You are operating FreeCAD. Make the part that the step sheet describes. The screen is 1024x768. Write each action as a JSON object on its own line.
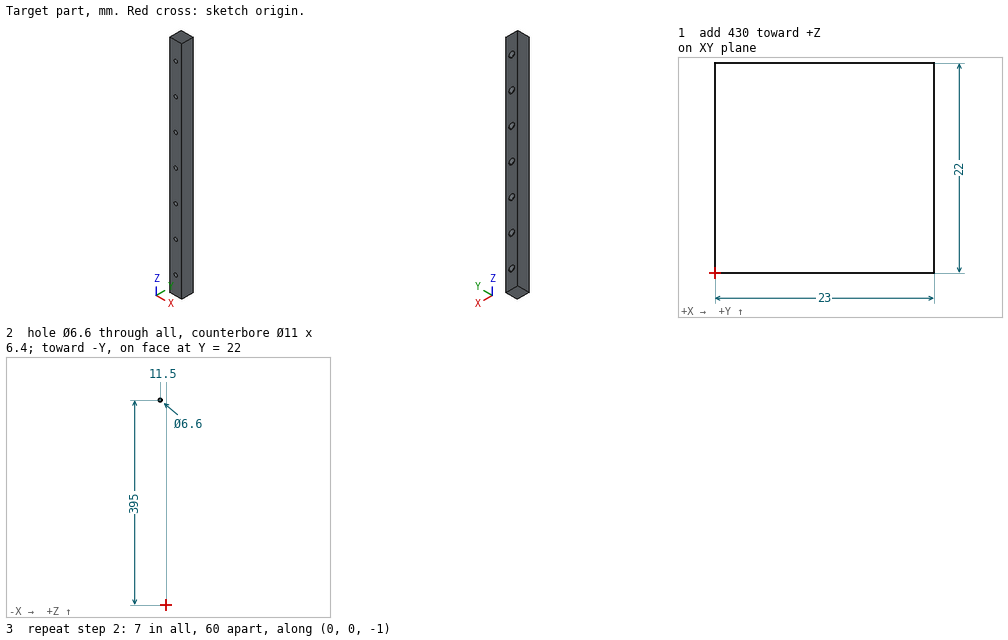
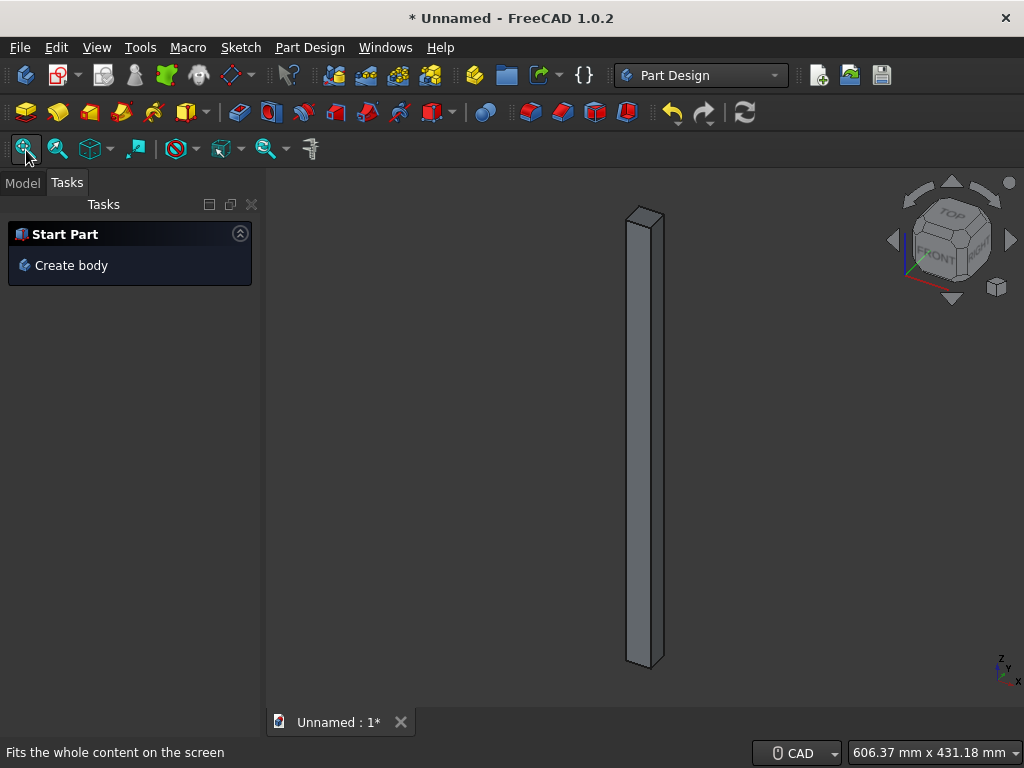
{"action": "key", "text": "4"}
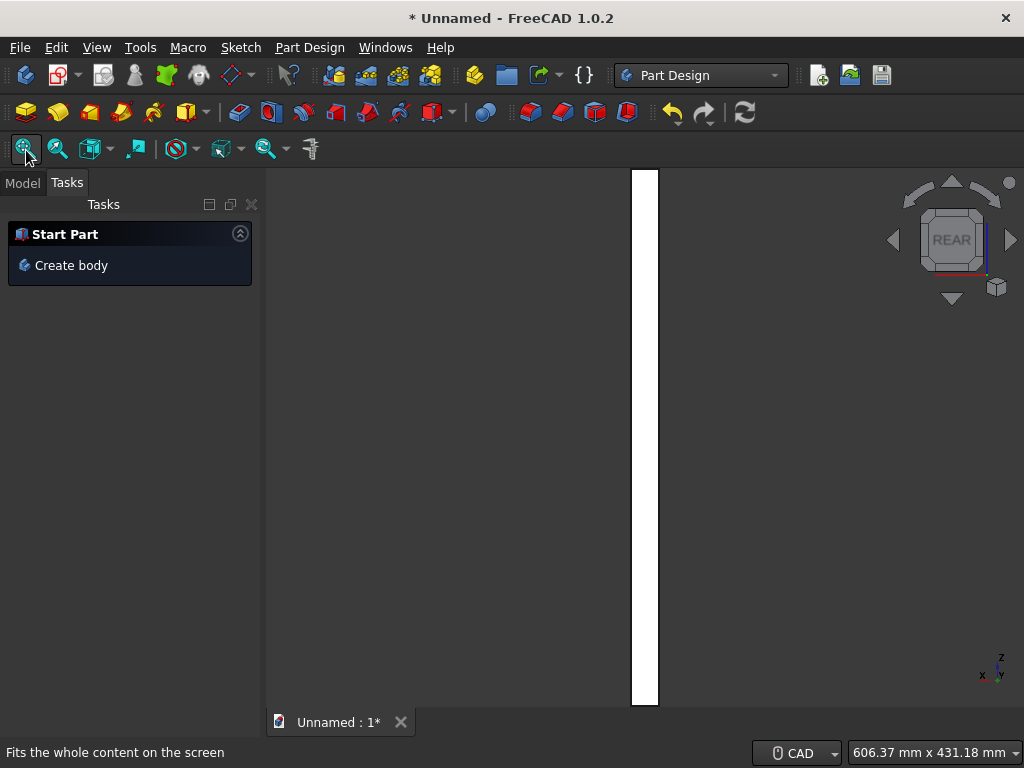
{"action": "left_click", "coordinate": [645, 206]}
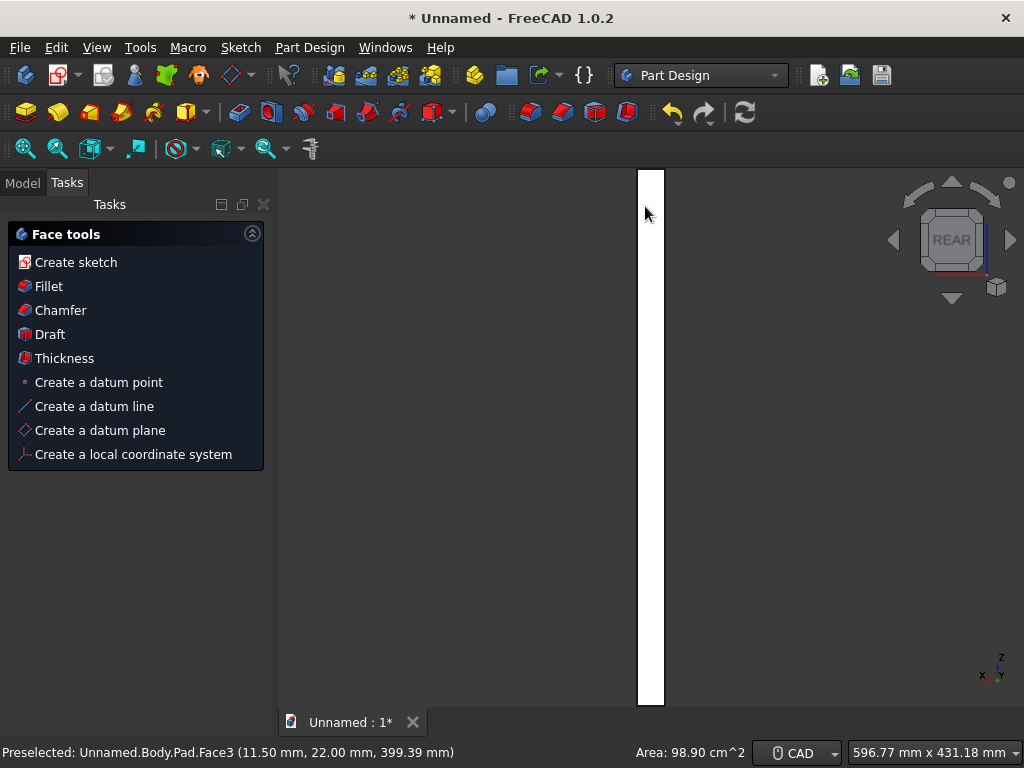
{"action": "left_click", "coordinate": [58, 76]}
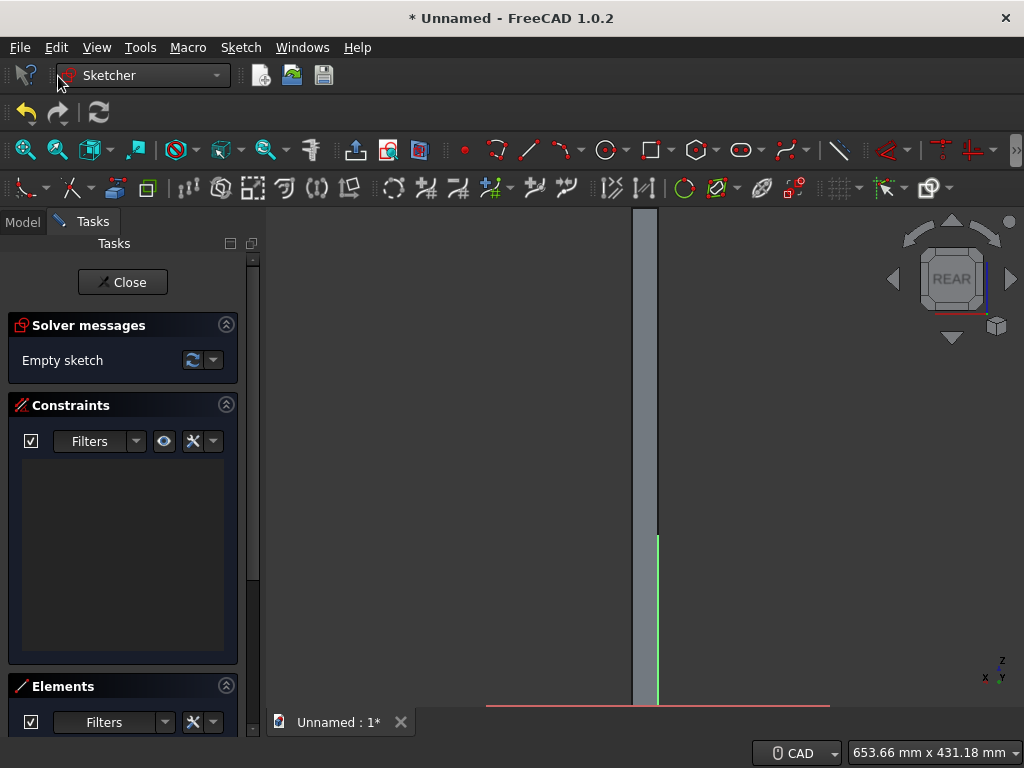
{"action": "scroll", "coordinate": [649, 237], "scroll_direction": "up", "scroll_amount": 15}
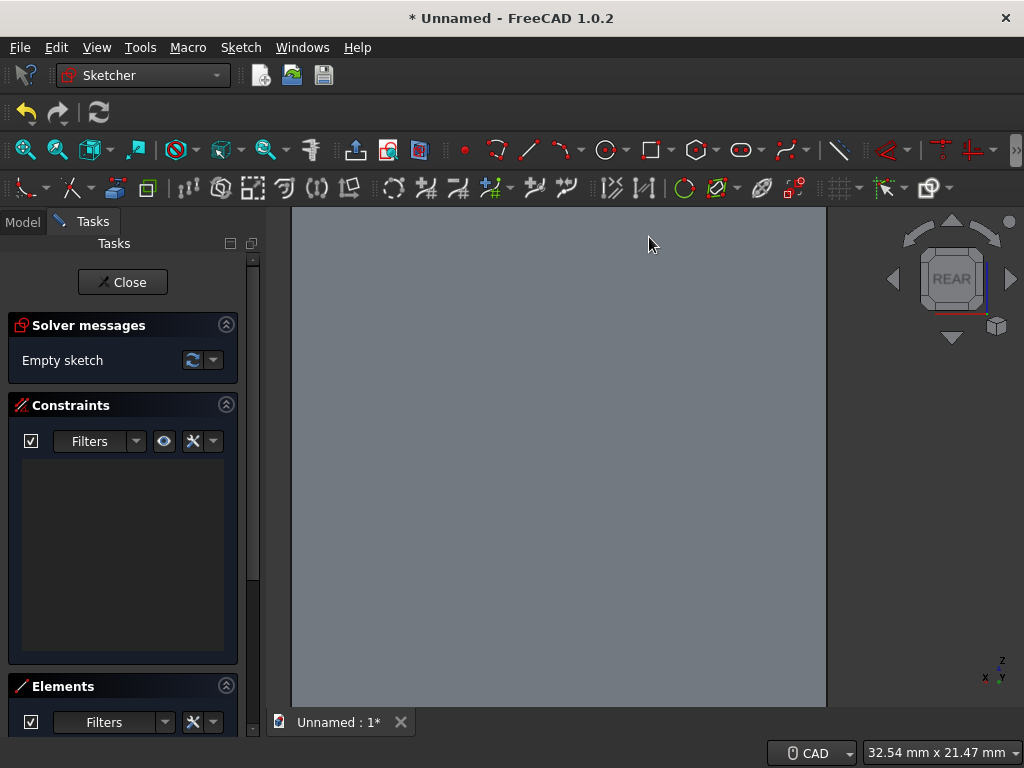
{"action": "scroll", "coordinate": [545, 466], "scroll_direction": "up", "scroll_amount": 4}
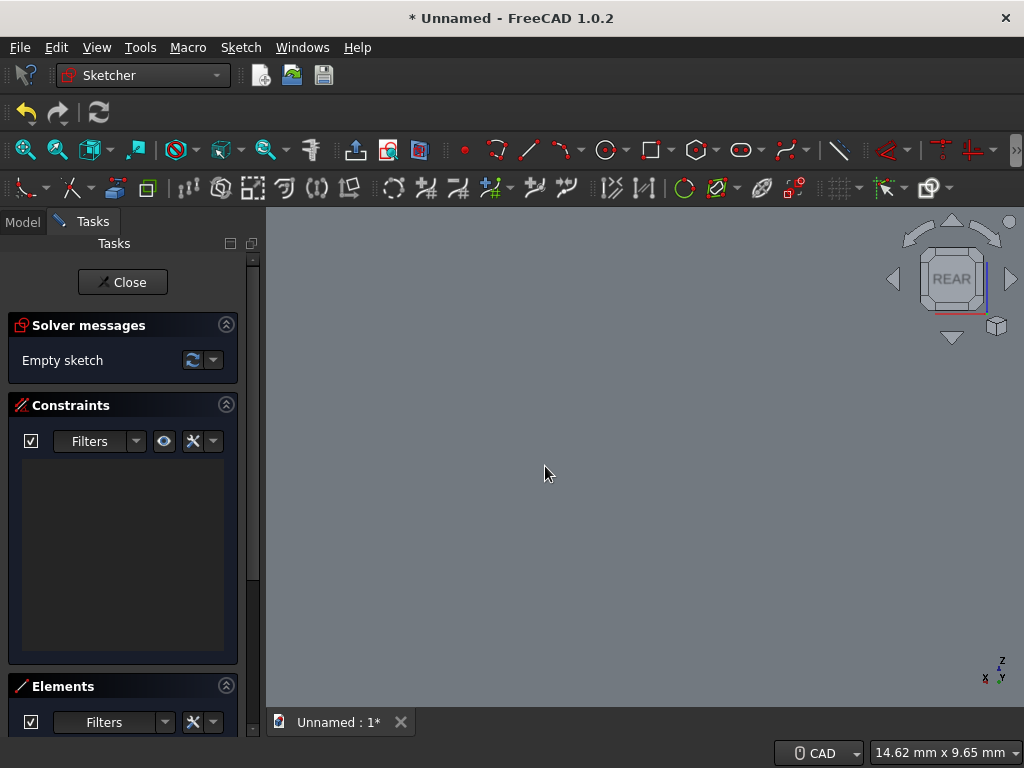
{"action": "left_click", "coordinate": [606, 150]}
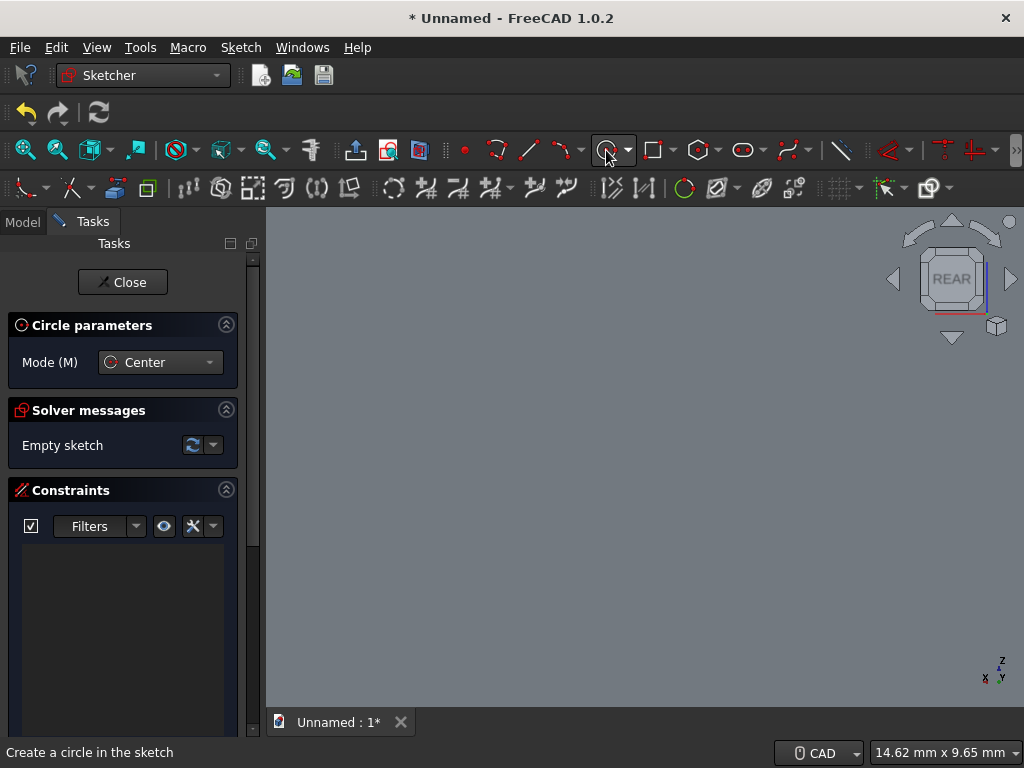
{"action": "left_click", "coordinate": [576, 457]}
{"action": "mouse_move", "coordinate": [697, 336]}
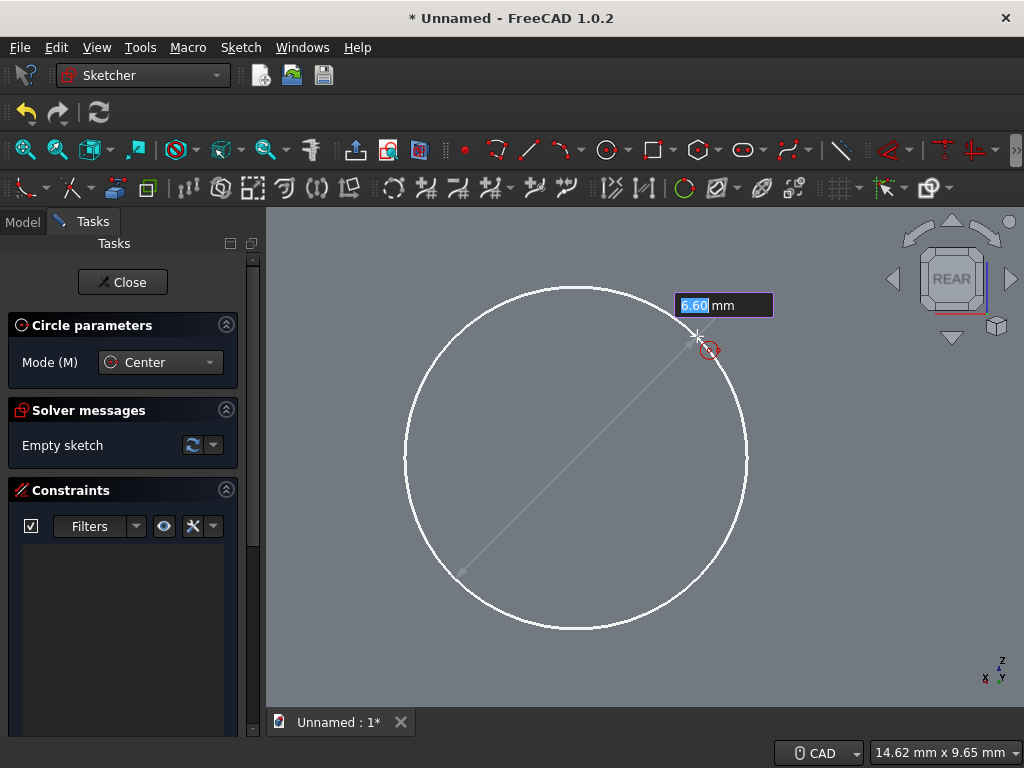
{"action": "type", "text": "6.6"}
{"action": "key", "text": "Return"}
{"action": "key", "text": "Escape"}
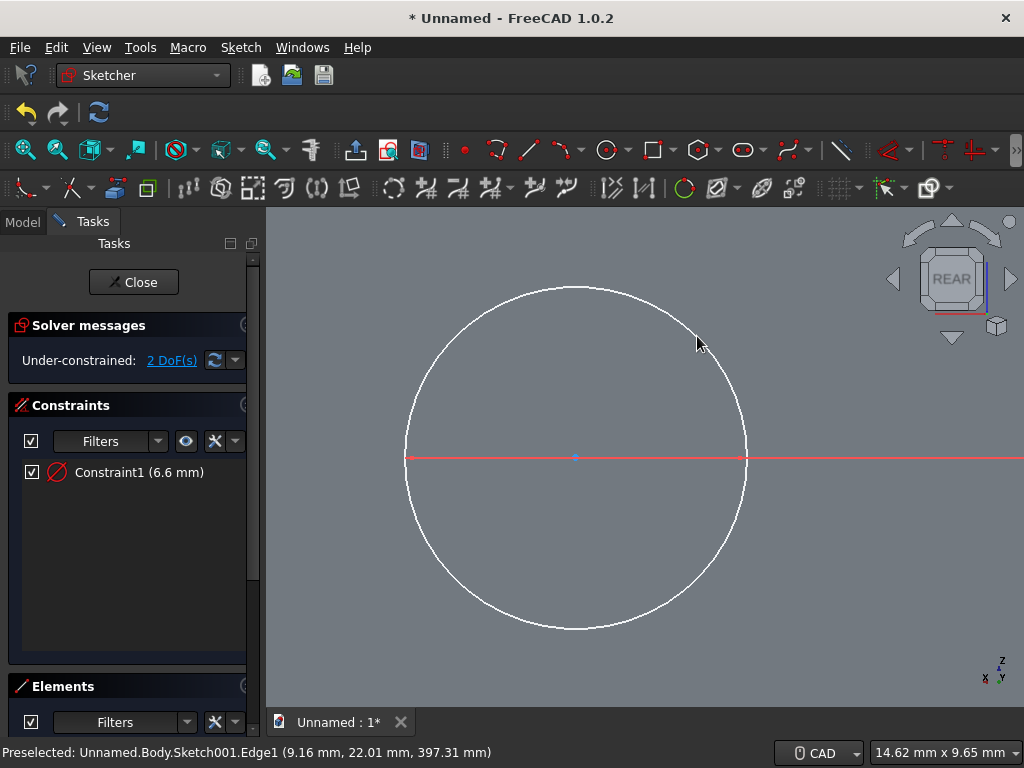
{"action": "left_click", "coordinate": [888, 150]}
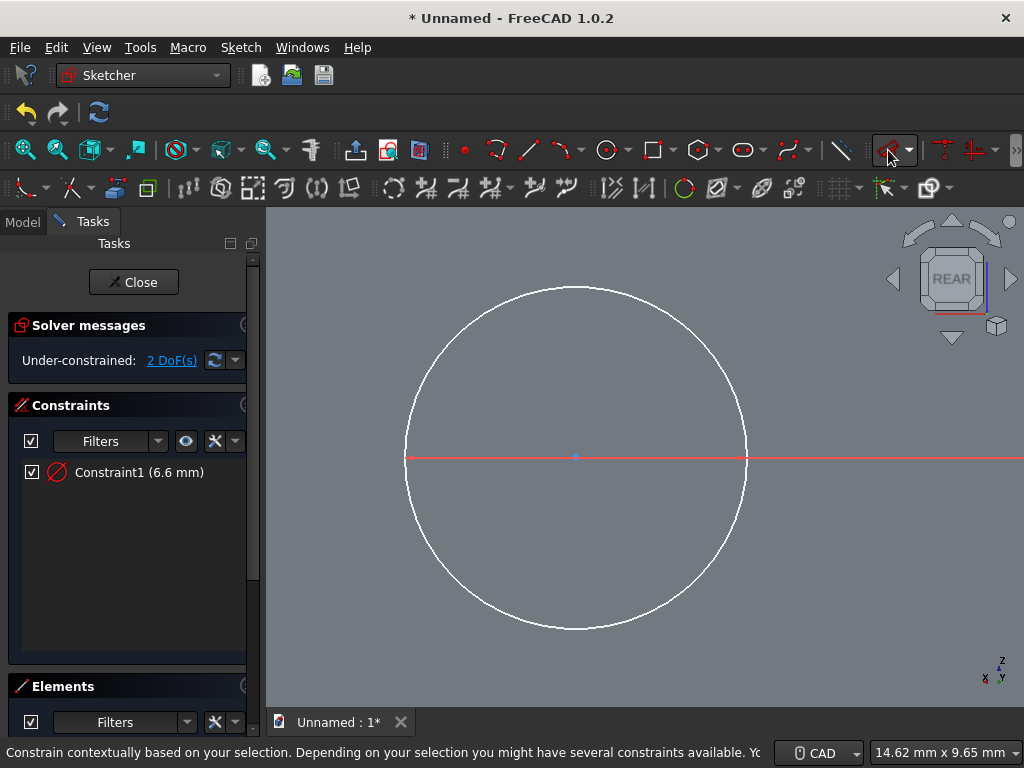
{"action": "left_click", "coordinate": [576, 458]}
{"action": "left_click", "coordinate": [542, 568]}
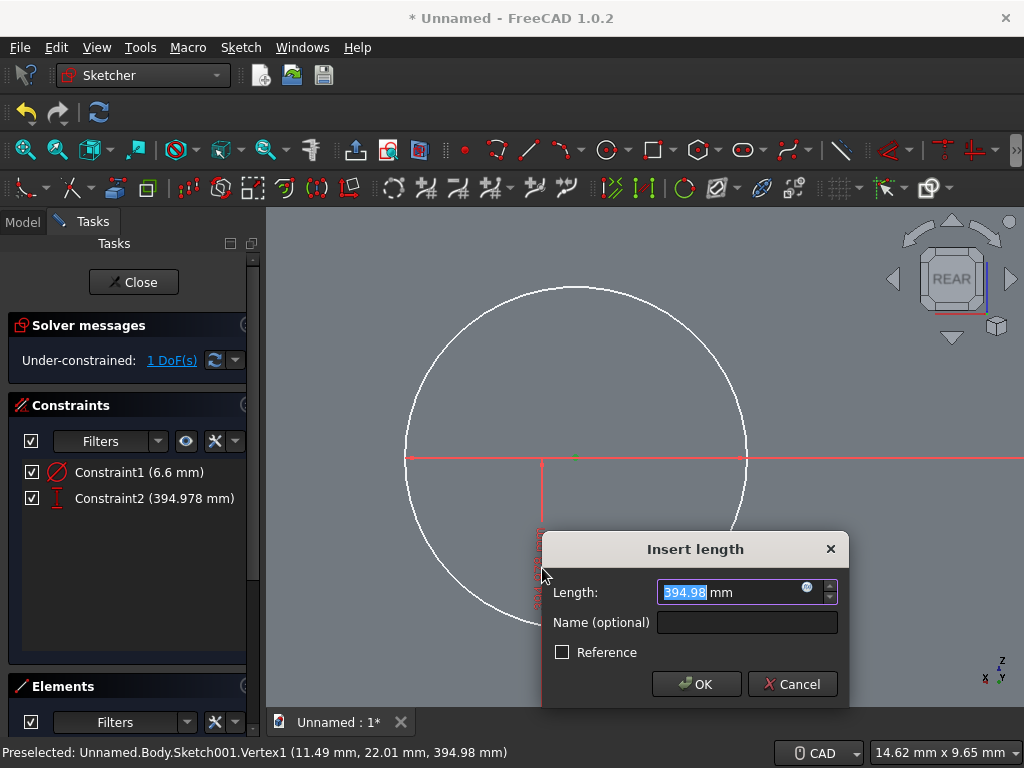
{"action": "type", "text": "395"}
{"action": "key", "text": "Return"}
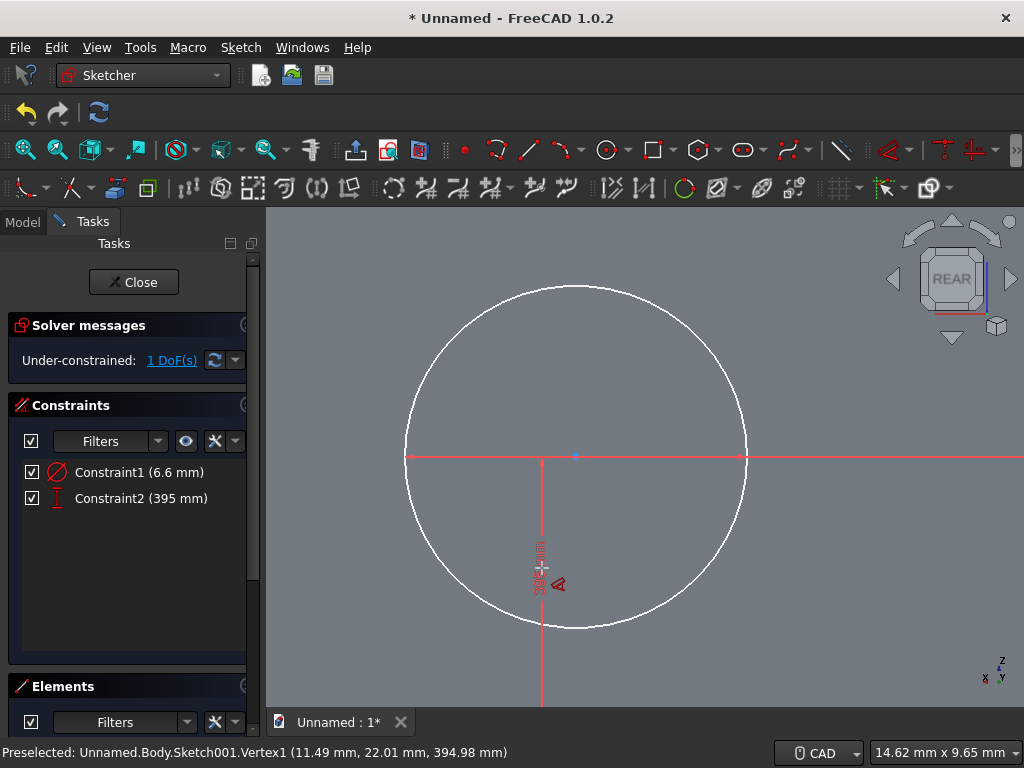
{"action": "left_click", "coordinate": [576, 457]}
{"action": "left_click", "coordinate": [717, 423]}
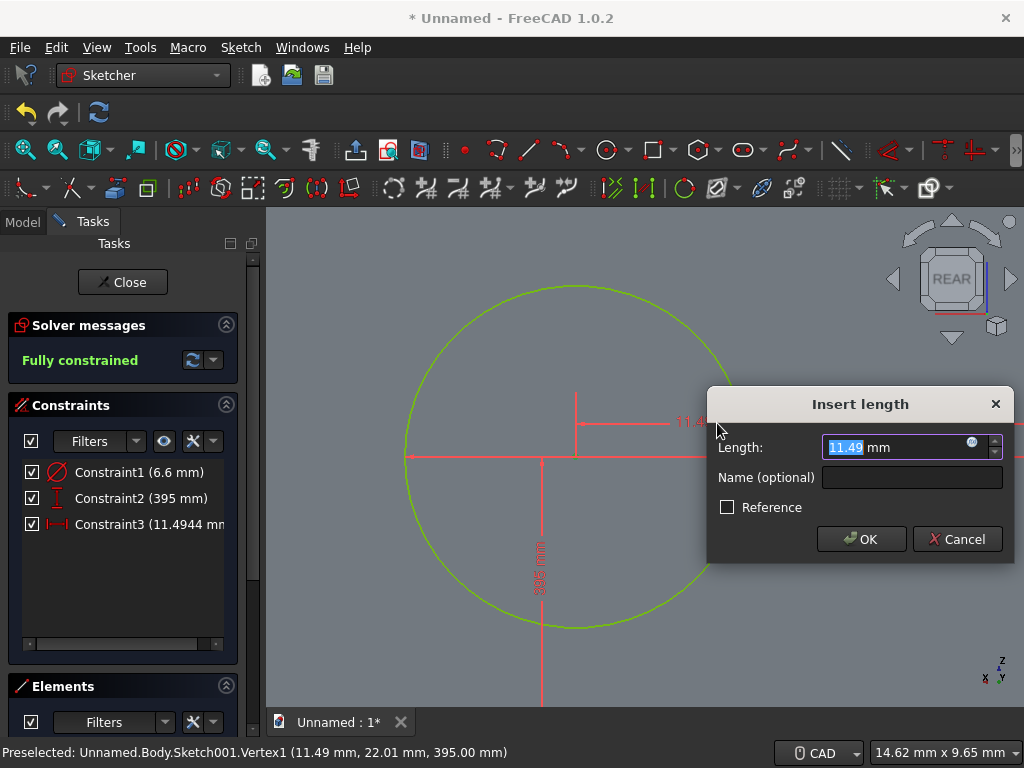
{"action": "type", "text": "11.5"}
{"action": "key", "text": "Return"}
{"action": "key", "text": "Escape"}